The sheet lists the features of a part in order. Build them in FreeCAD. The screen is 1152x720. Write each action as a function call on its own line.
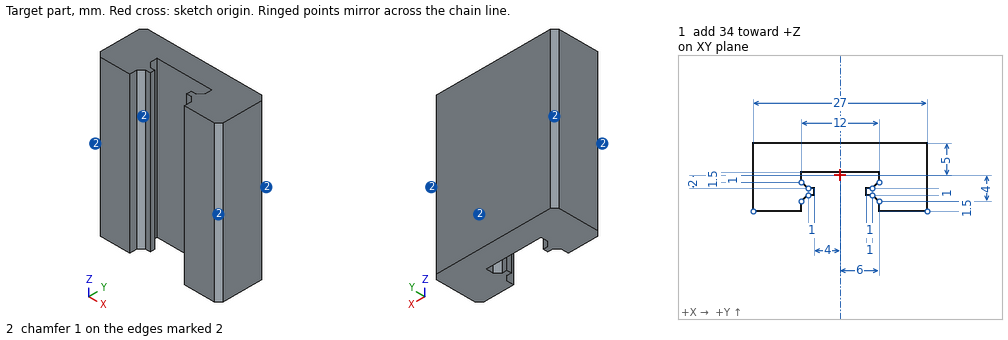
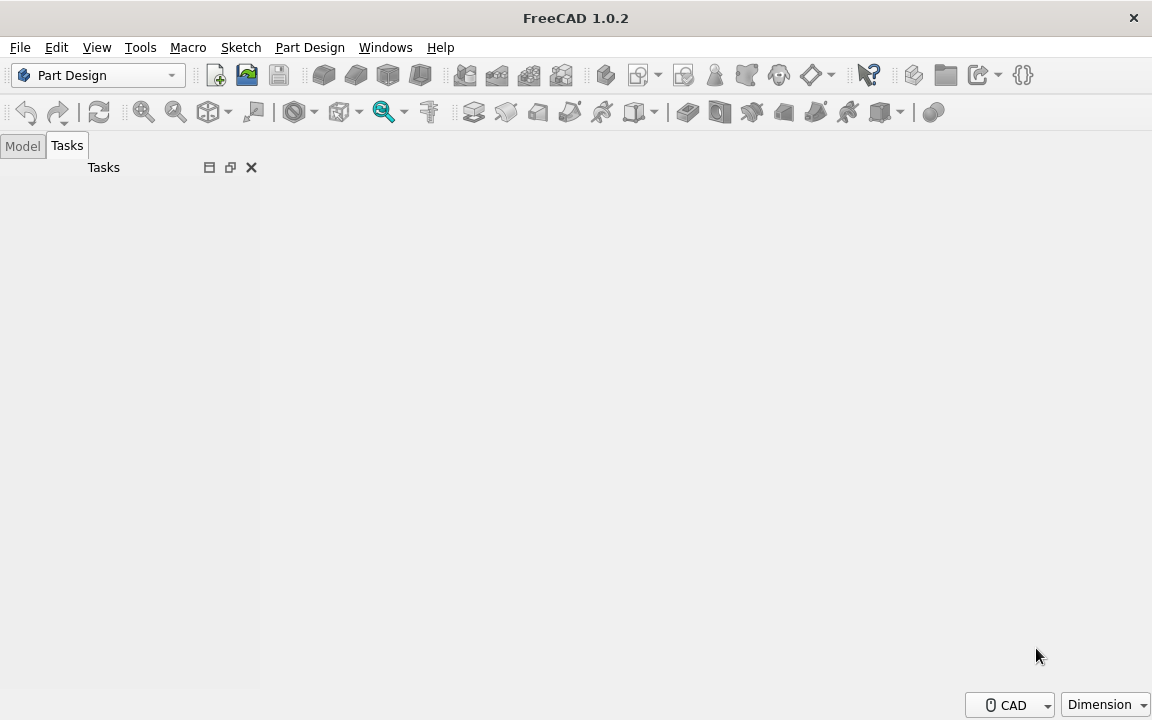
click(216, 76)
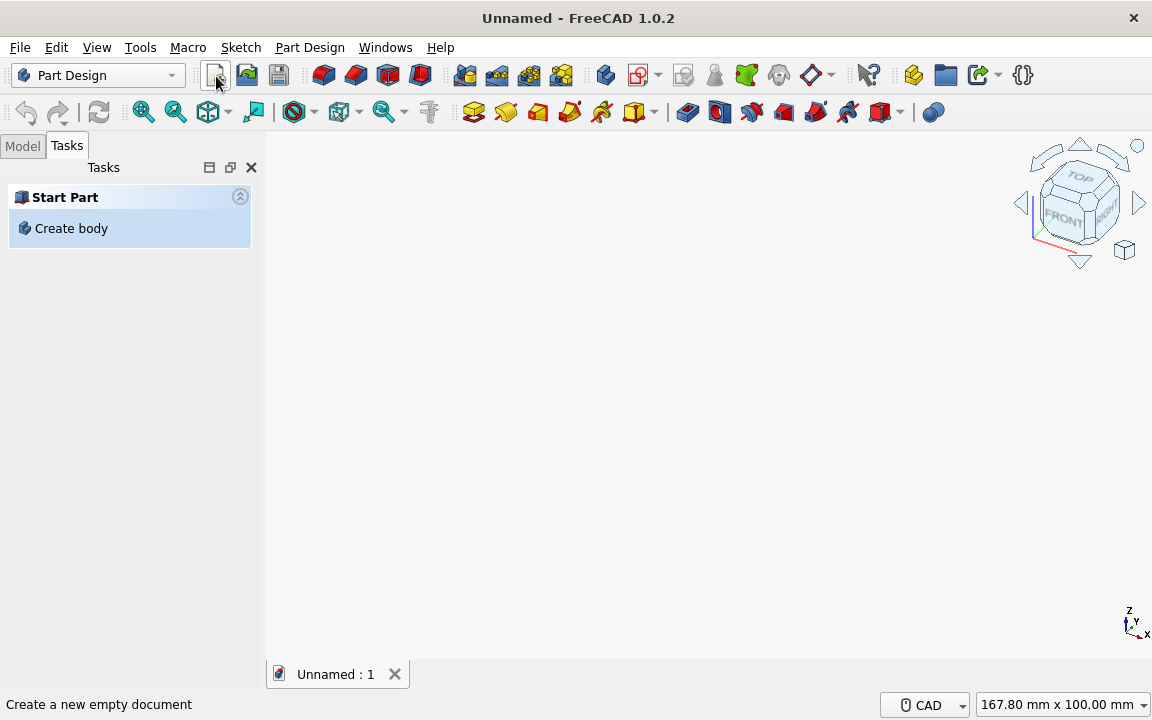
click(638, 76)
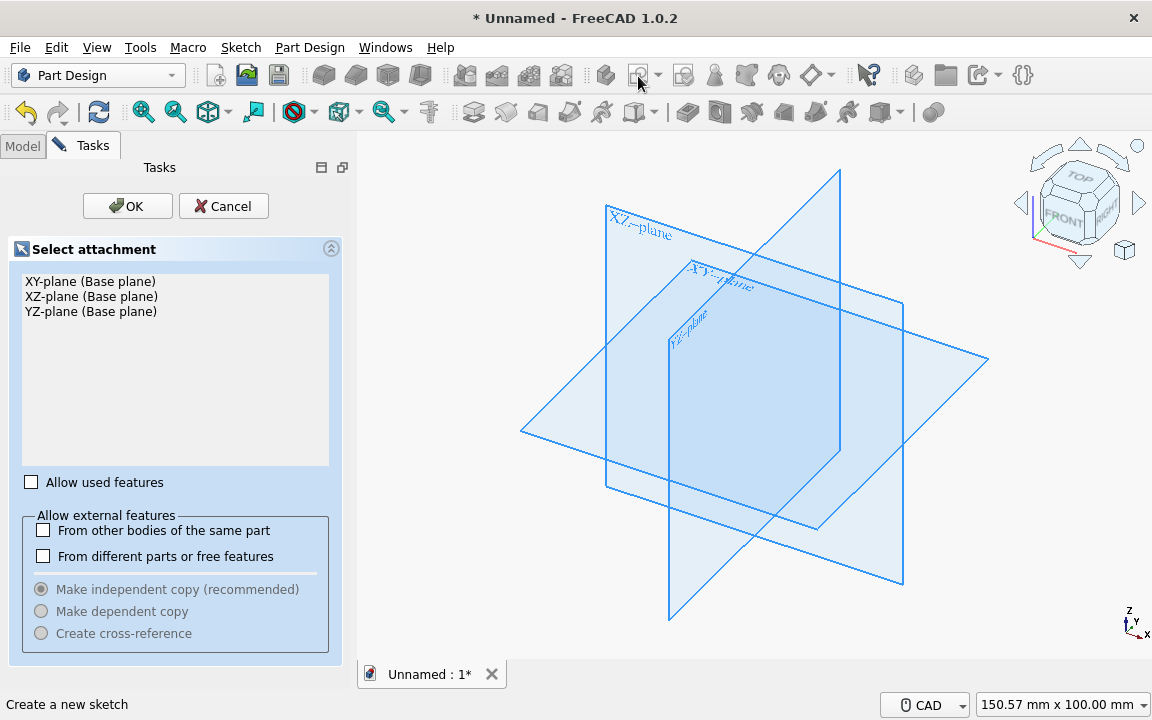
click(82, 282)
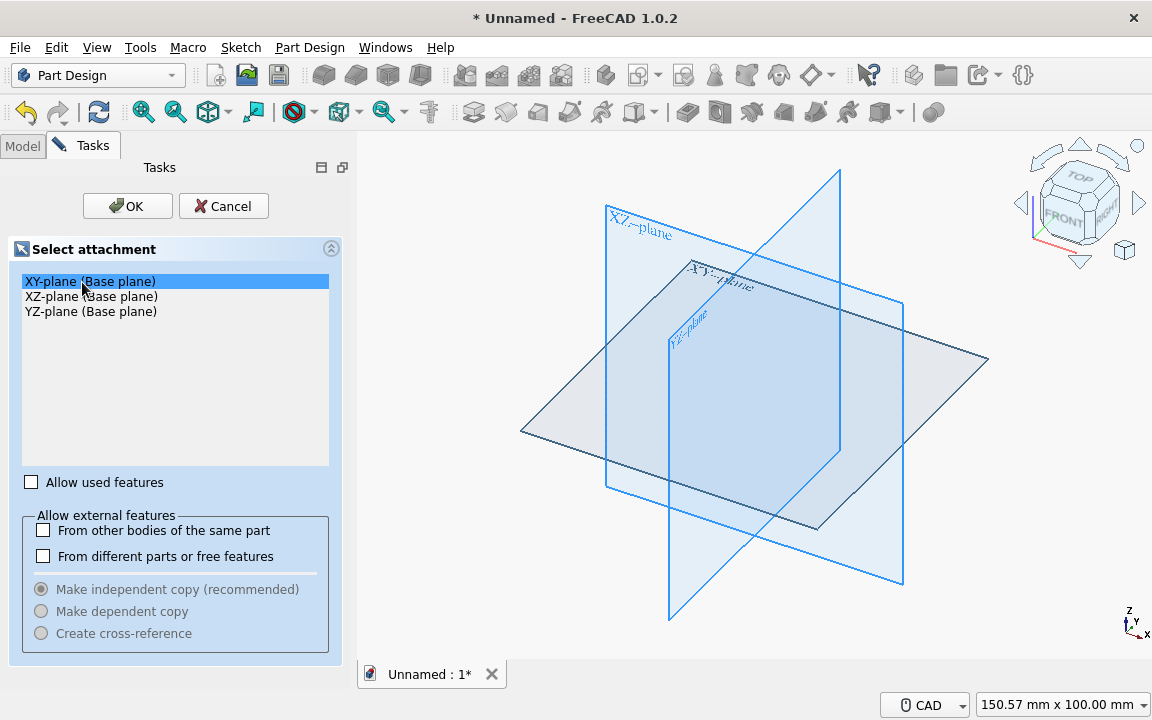
click(128, 206)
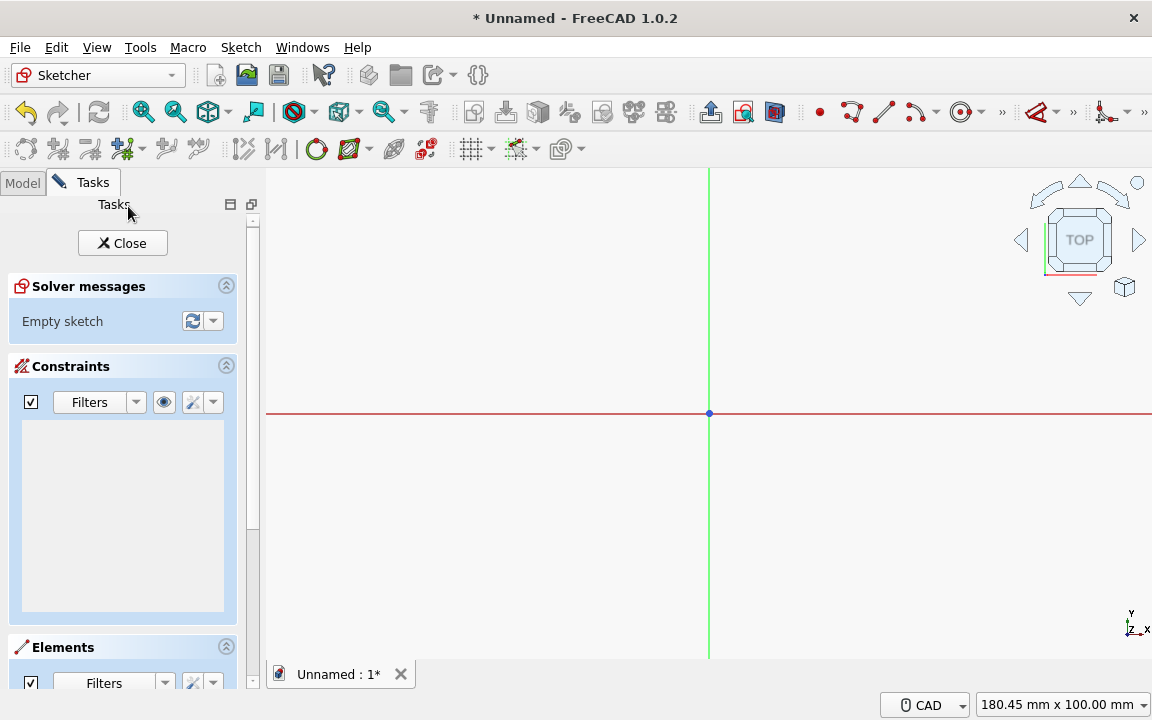
scroll(731, 415, up, 7)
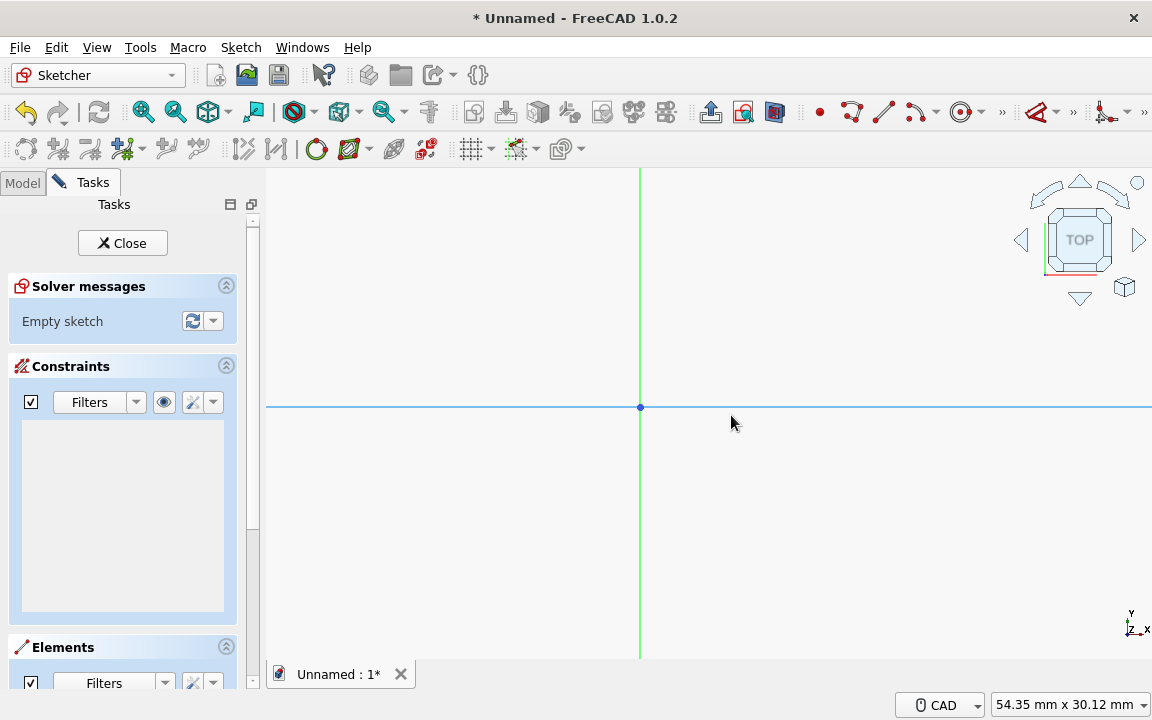
click(852, 112)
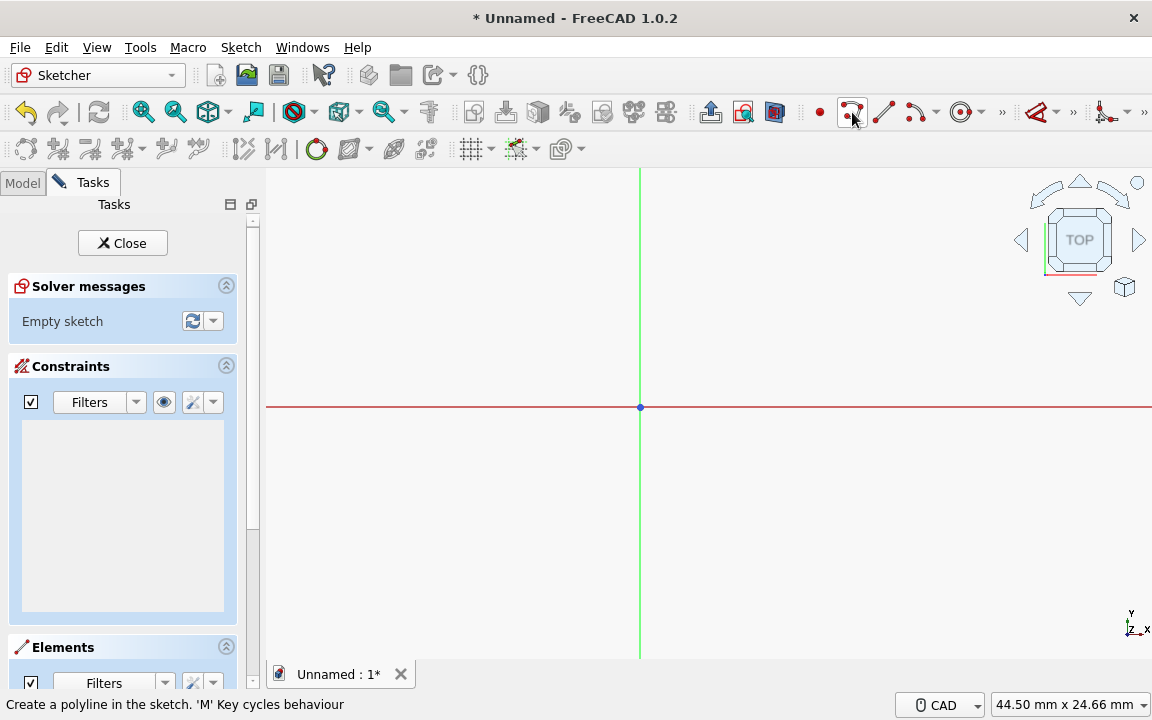
click(561, 447)
click(541, 447)
click(521, 427)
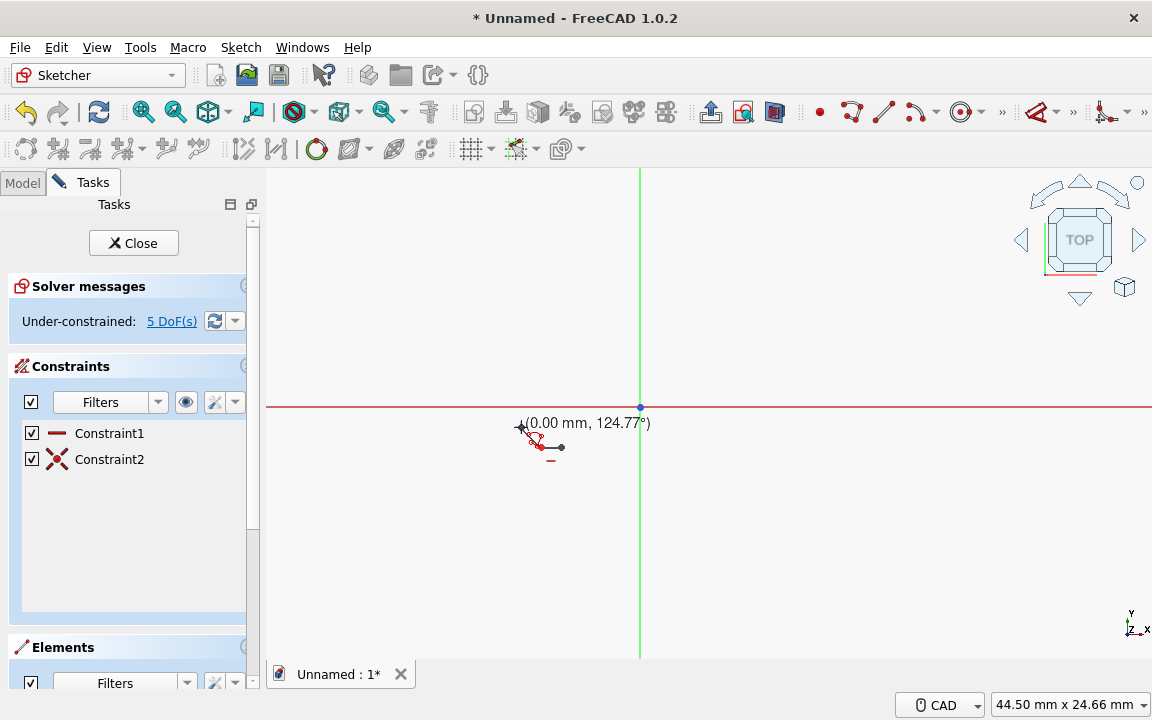
scroll(521, 397, up, 3)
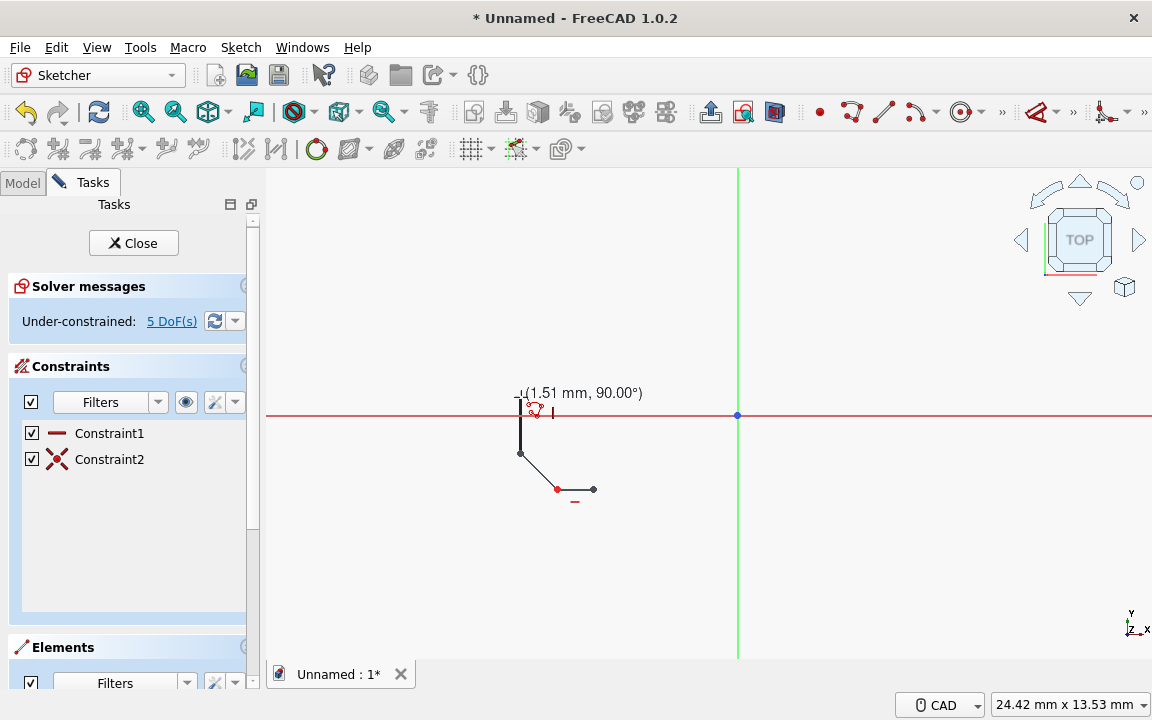
click(521, 397)
click(956, 397)
click(956, 452)
click(919, 488)
click(883, 488)
click(883, 524)
click(919, 524)
click(956, 561)
click(956, 615)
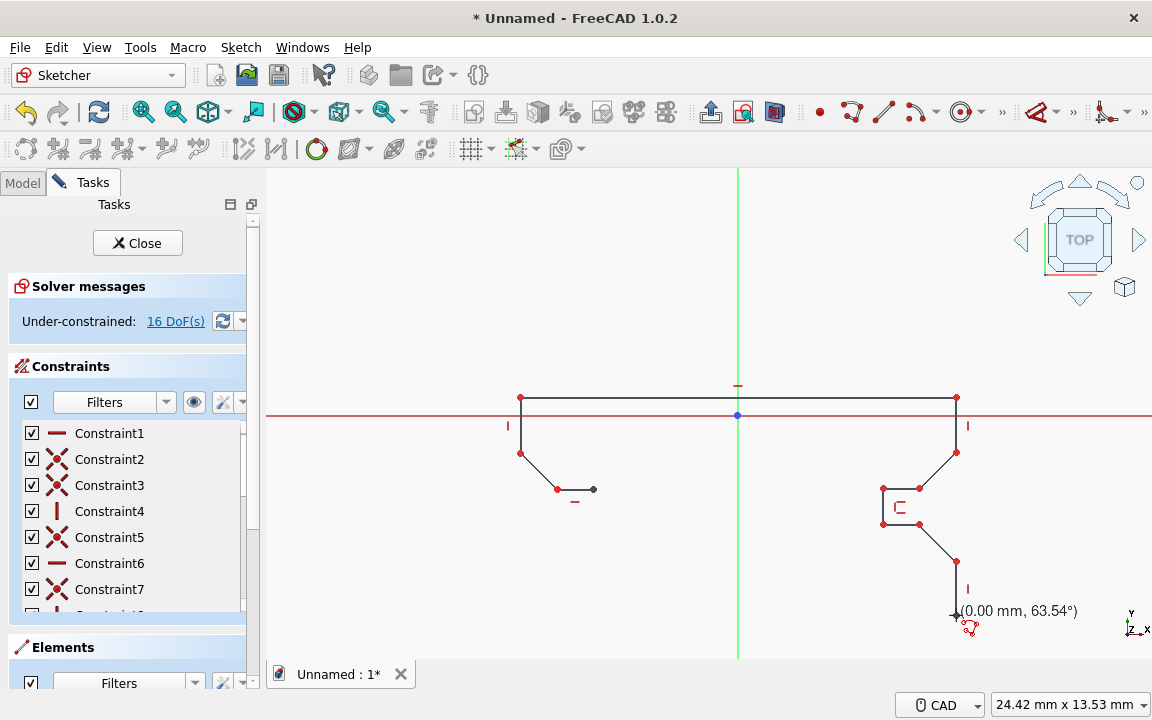
scroll(522, 400, down, 3)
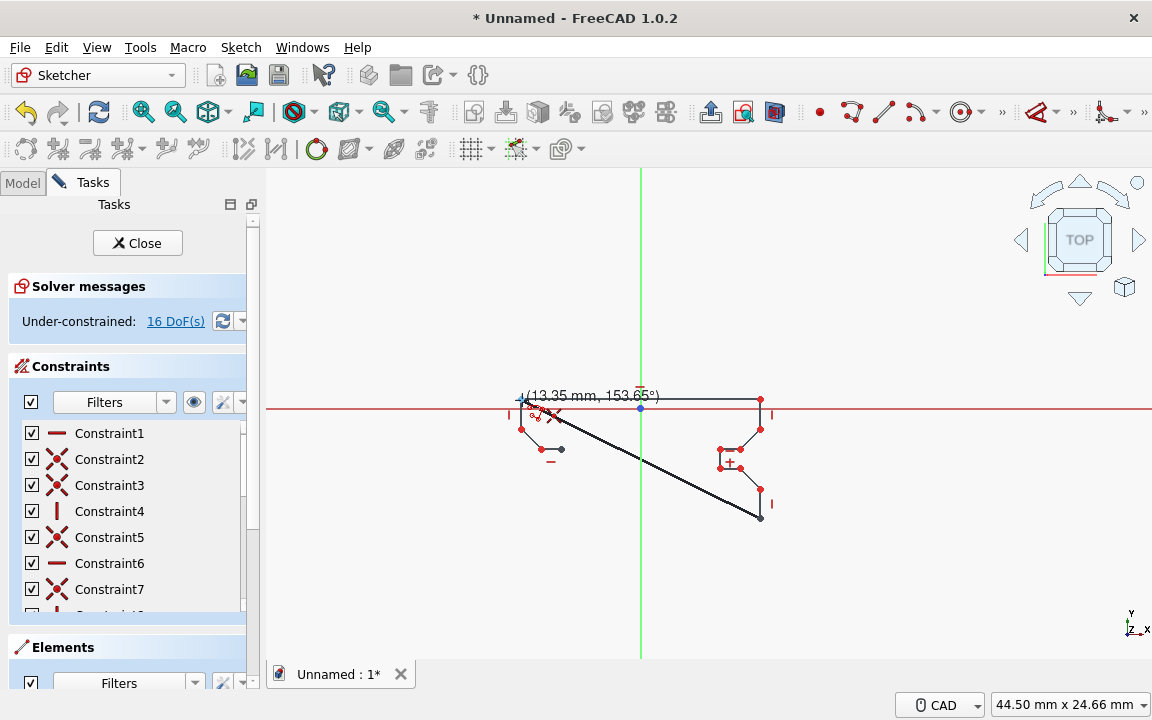
click(909, 518)
click(909, 309)
click(372, 309)
click(372, 518)
click(521, 518)
click(521, 488)
click(541, 468)
click(561, 468)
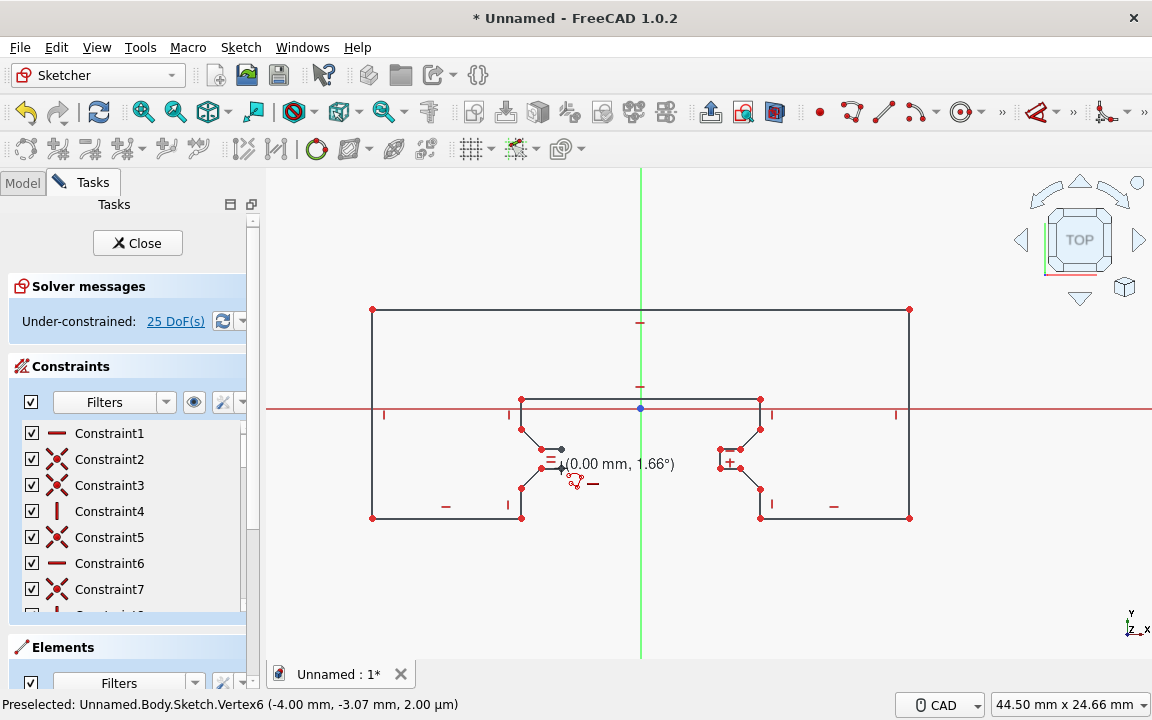
scroll(561, 449, up, 3)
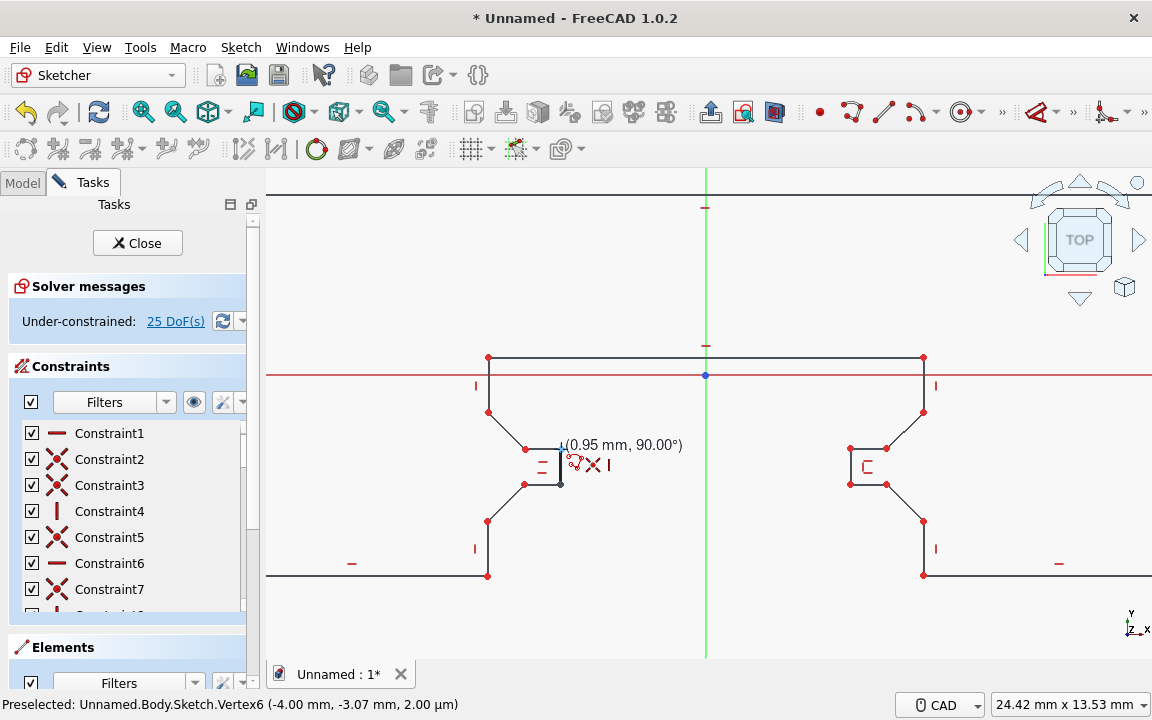
click(562, 449)
key(Escape)
key(Escape)